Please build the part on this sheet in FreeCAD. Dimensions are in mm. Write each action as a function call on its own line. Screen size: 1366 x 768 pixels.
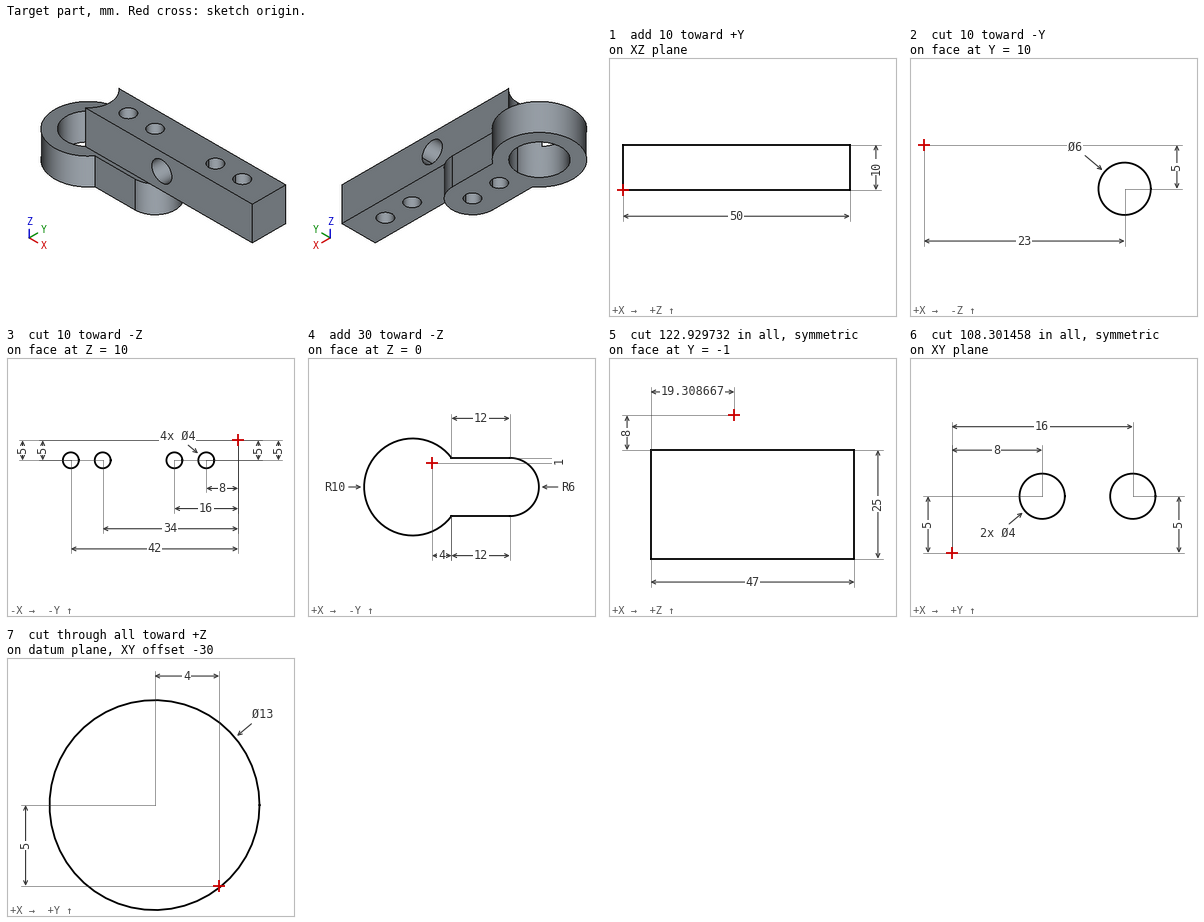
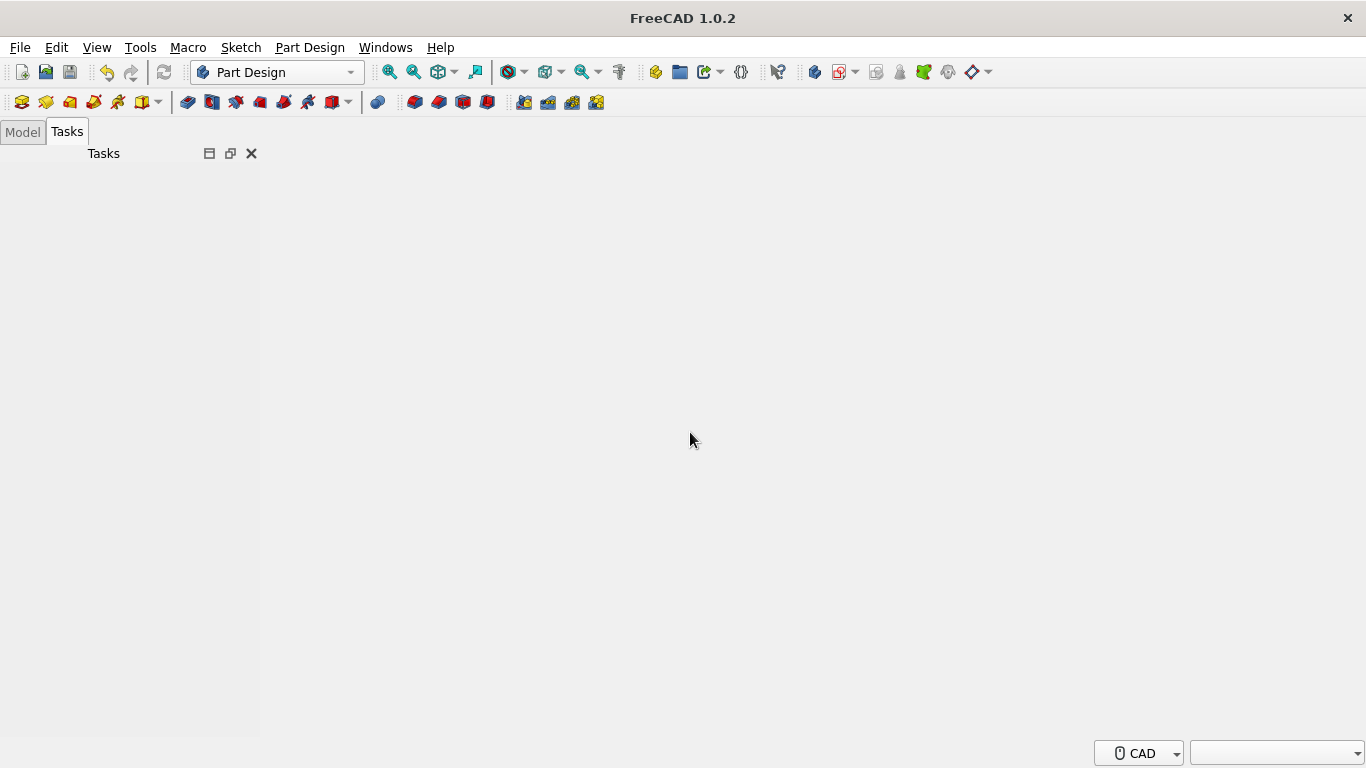
key(ctrl+n)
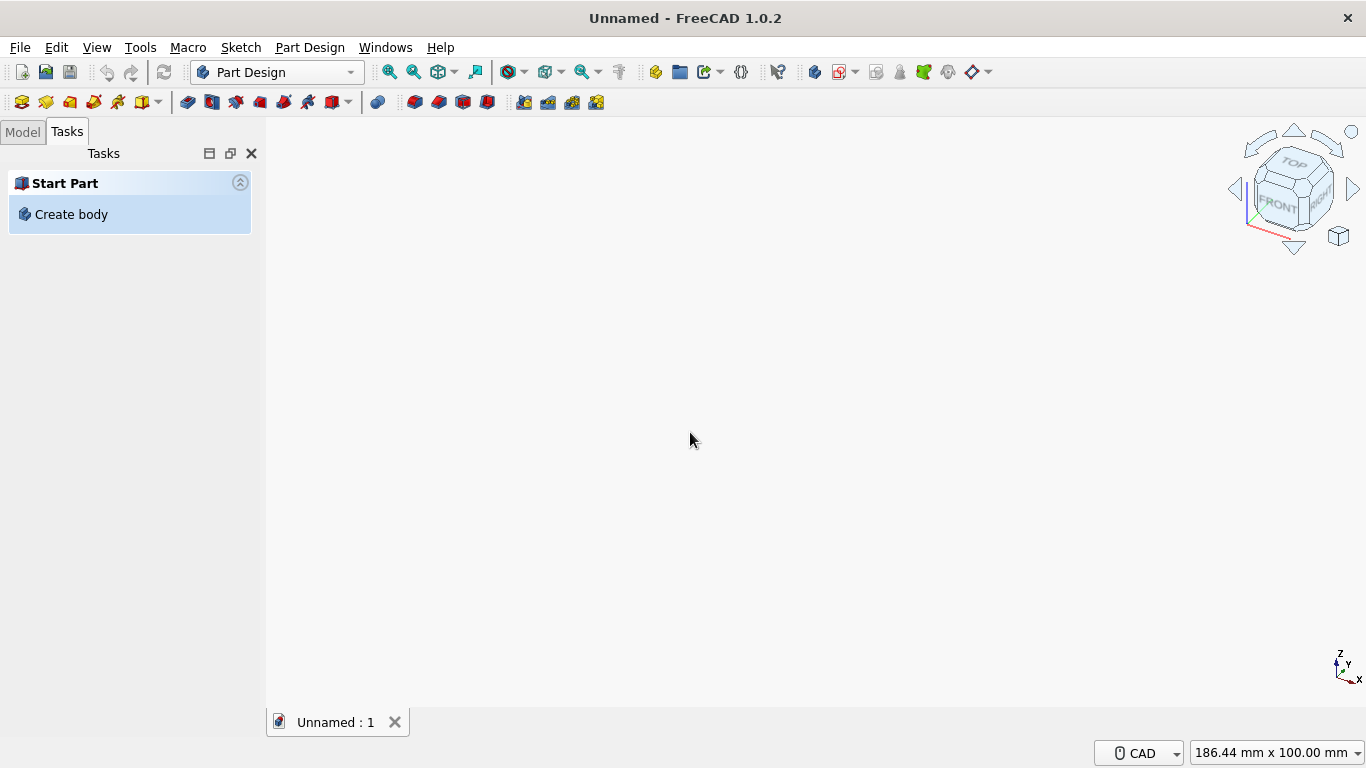
click(840, 72)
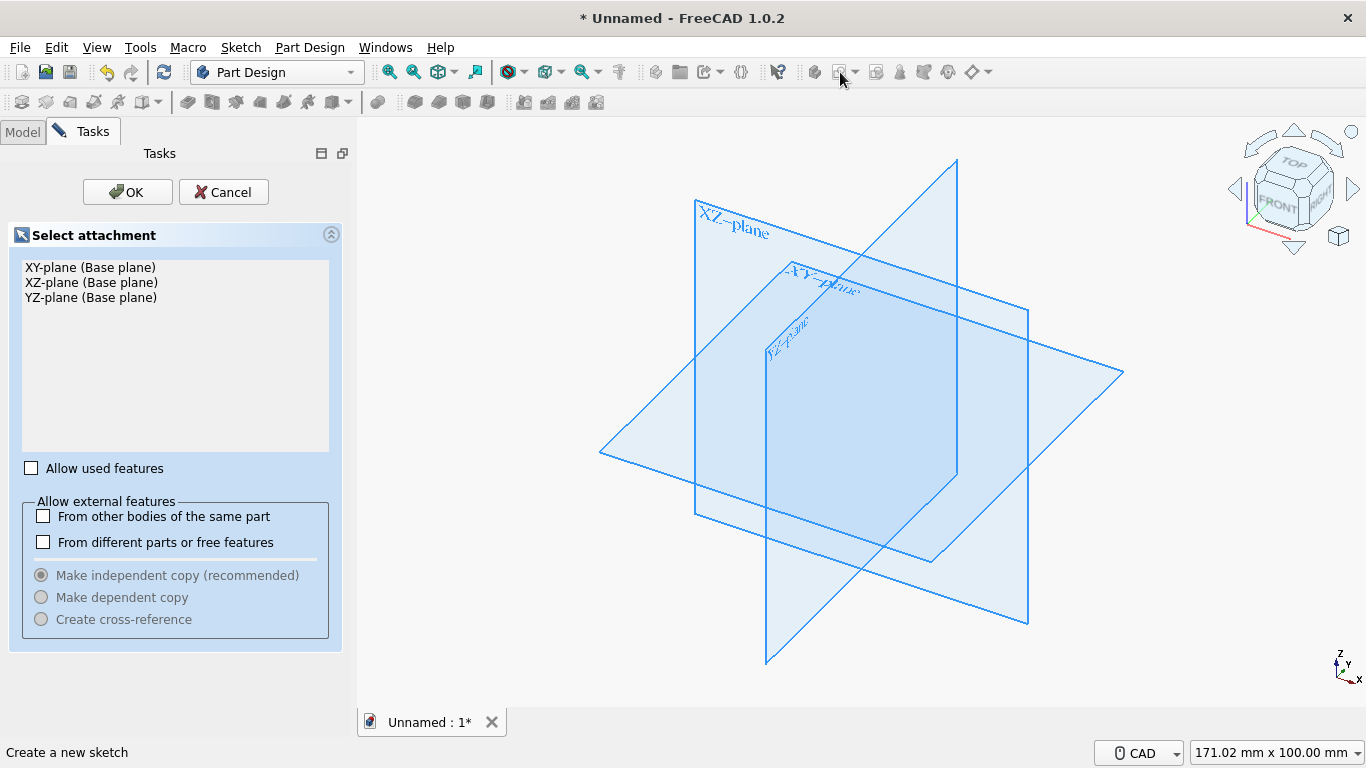
click(82, 282)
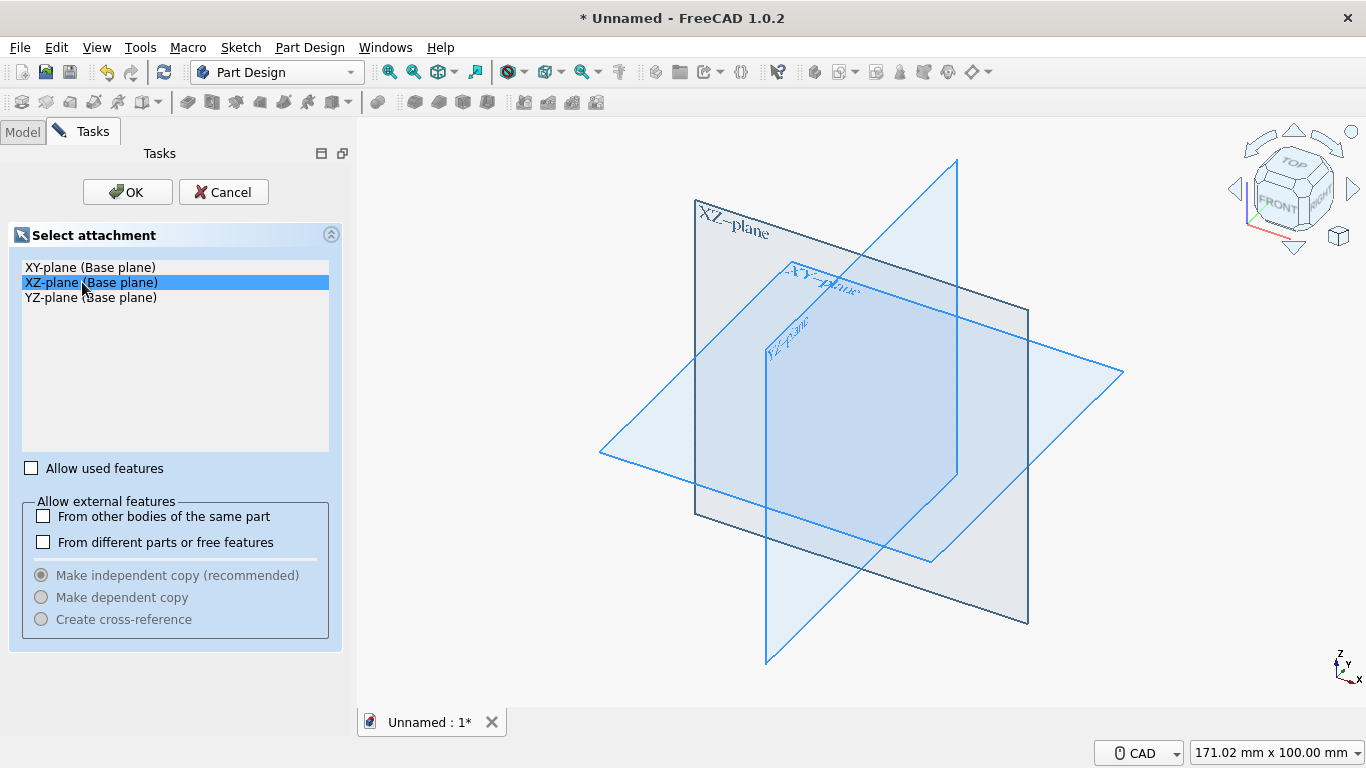
click(128, 192)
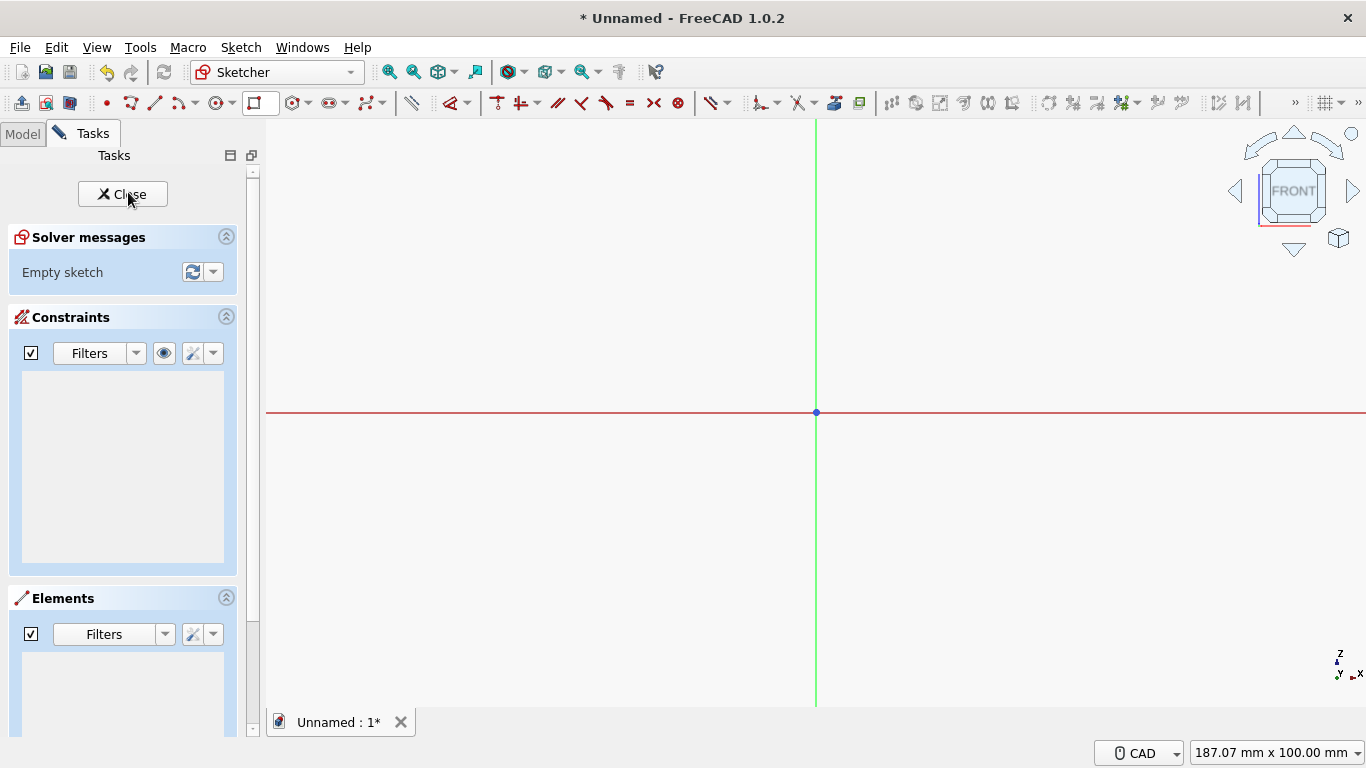
scroll(1139, 360, up, 4)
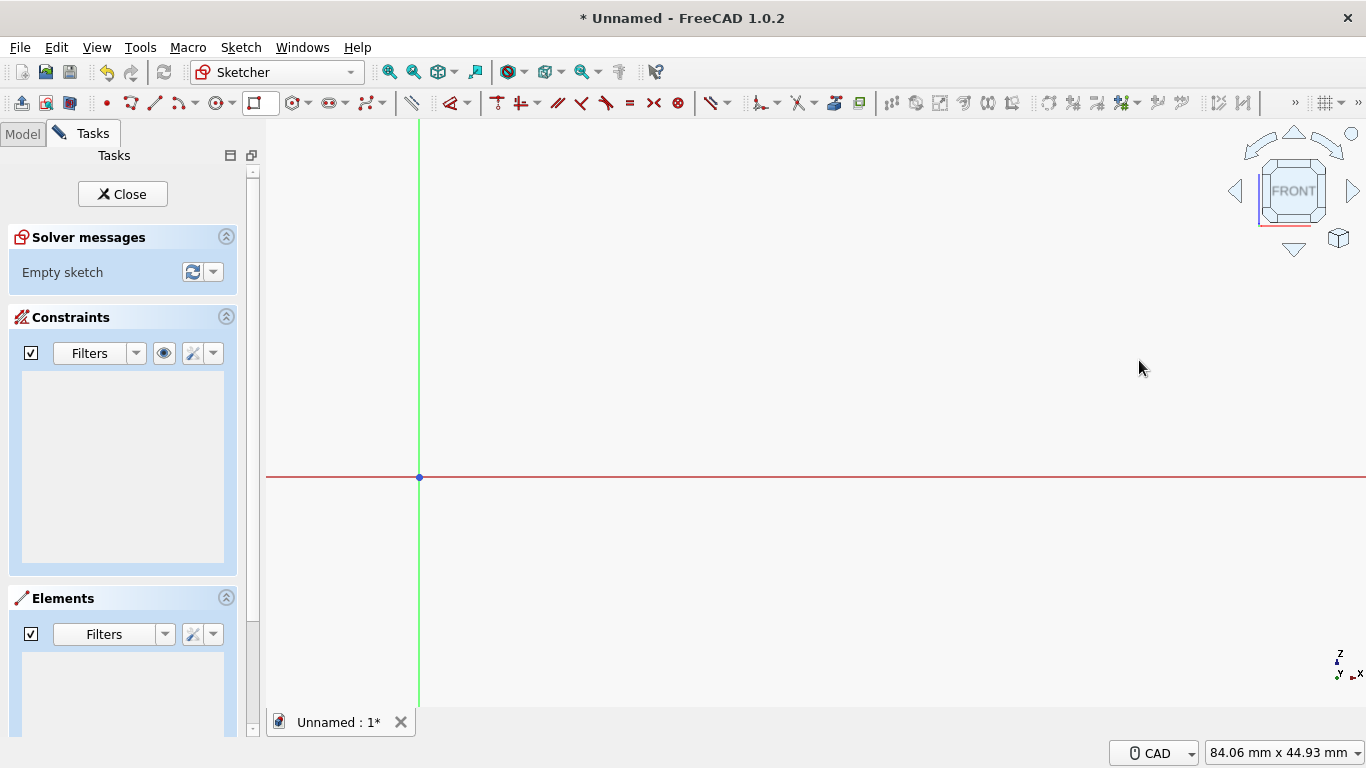
click(254, 104)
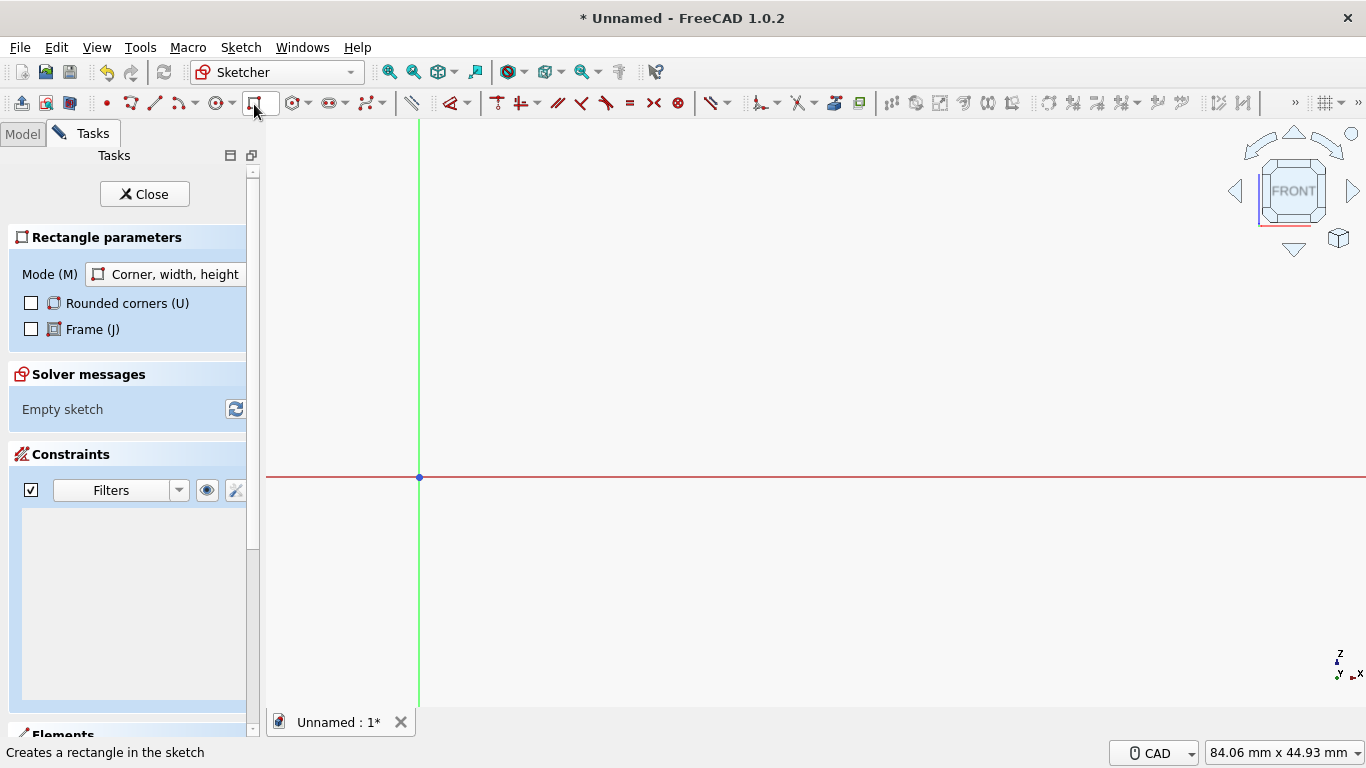
click(419, 477)
move(1073, 347)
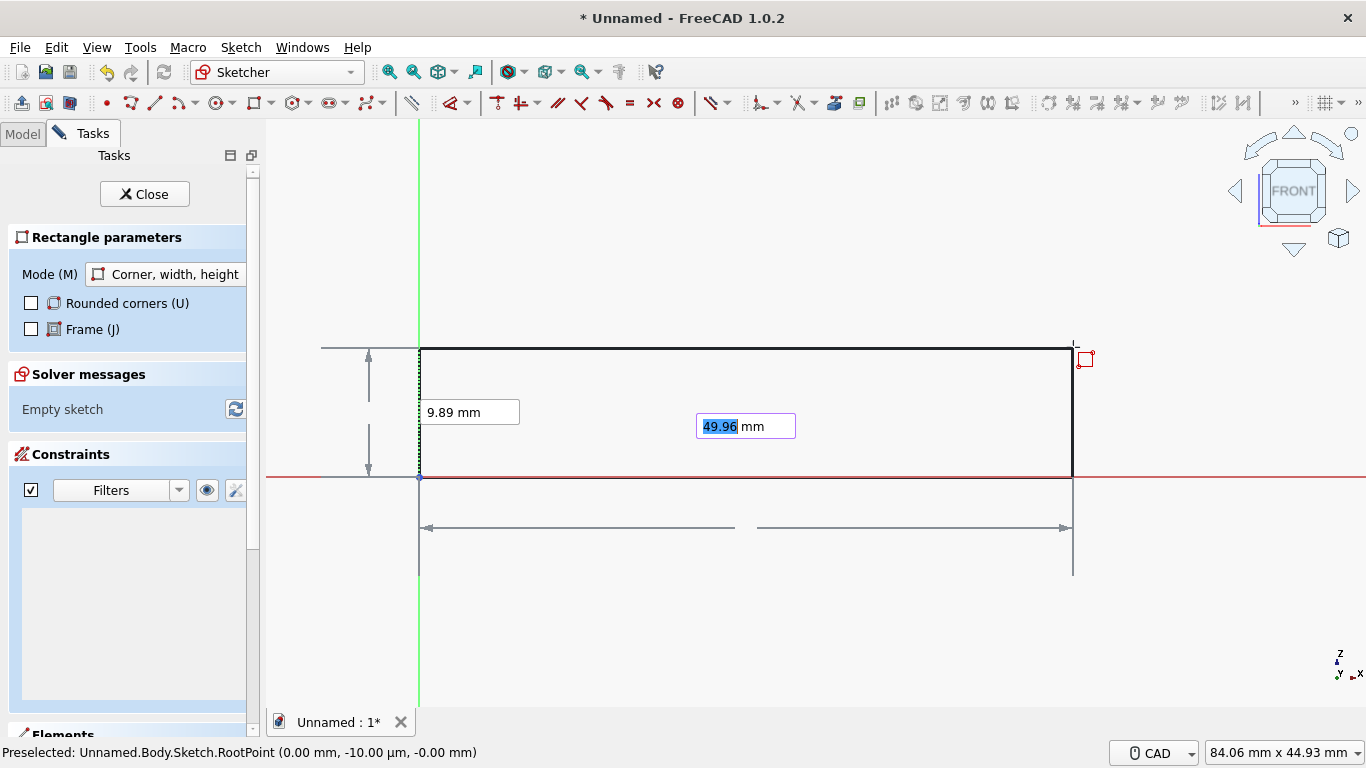
text(50)
key(Tab)
text(10)
key(Return)
key(Escape)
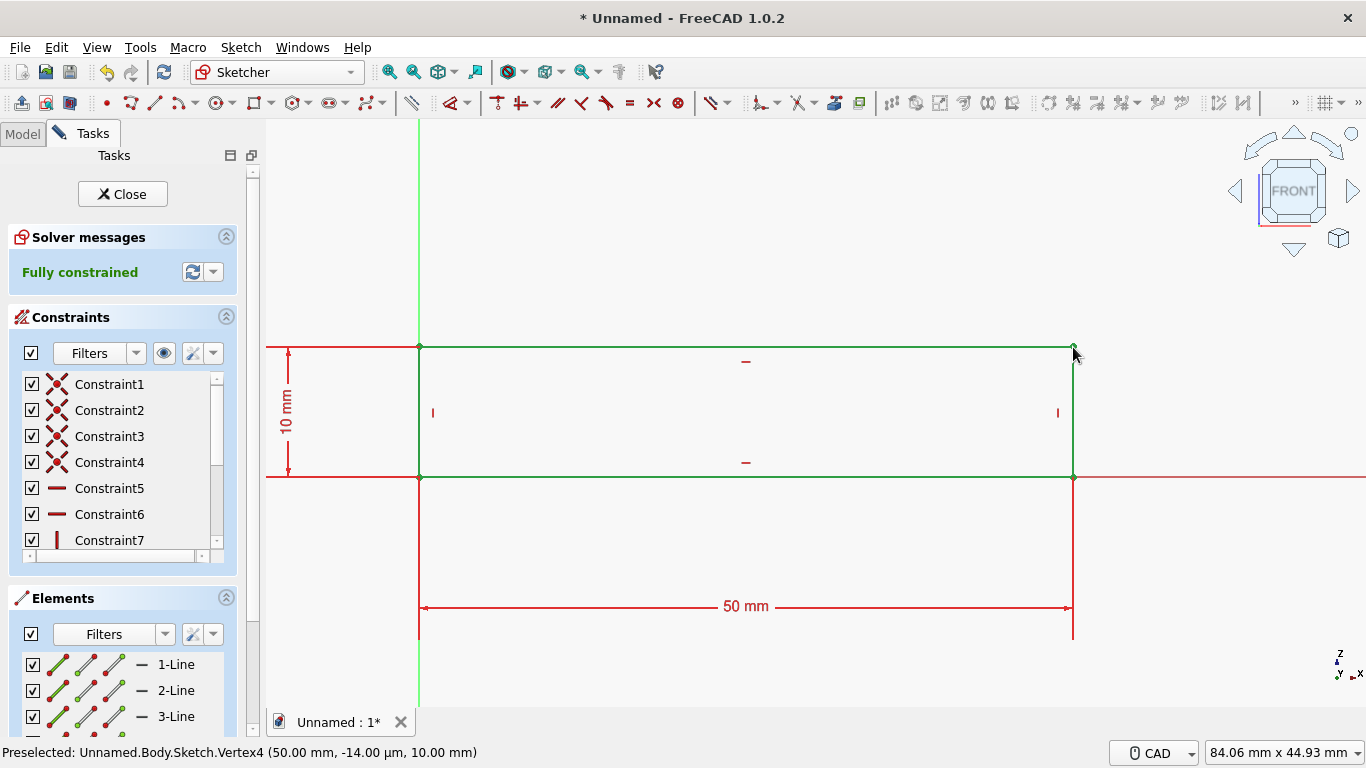
click(123, 194)